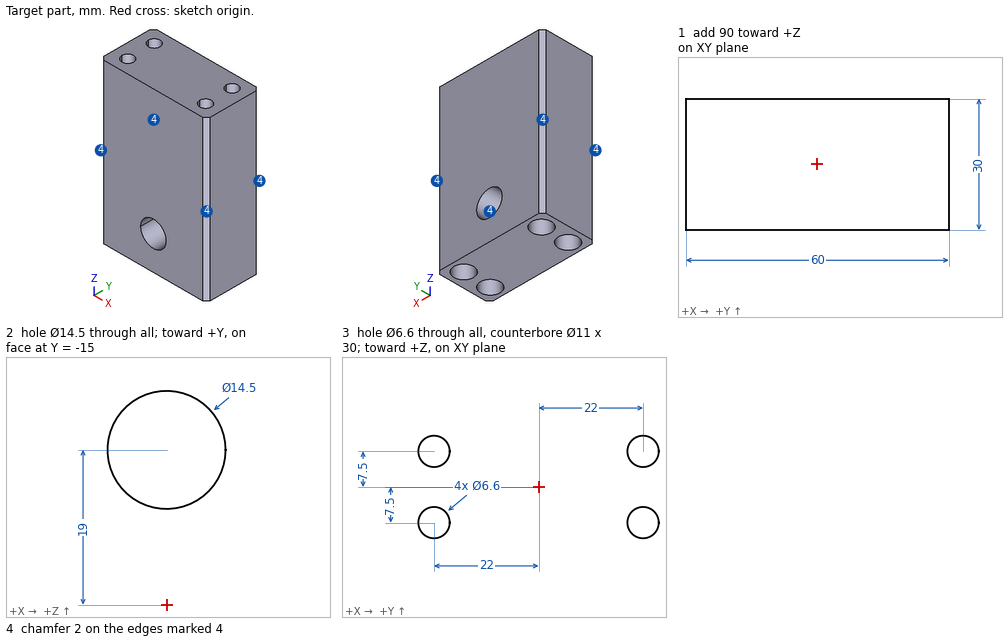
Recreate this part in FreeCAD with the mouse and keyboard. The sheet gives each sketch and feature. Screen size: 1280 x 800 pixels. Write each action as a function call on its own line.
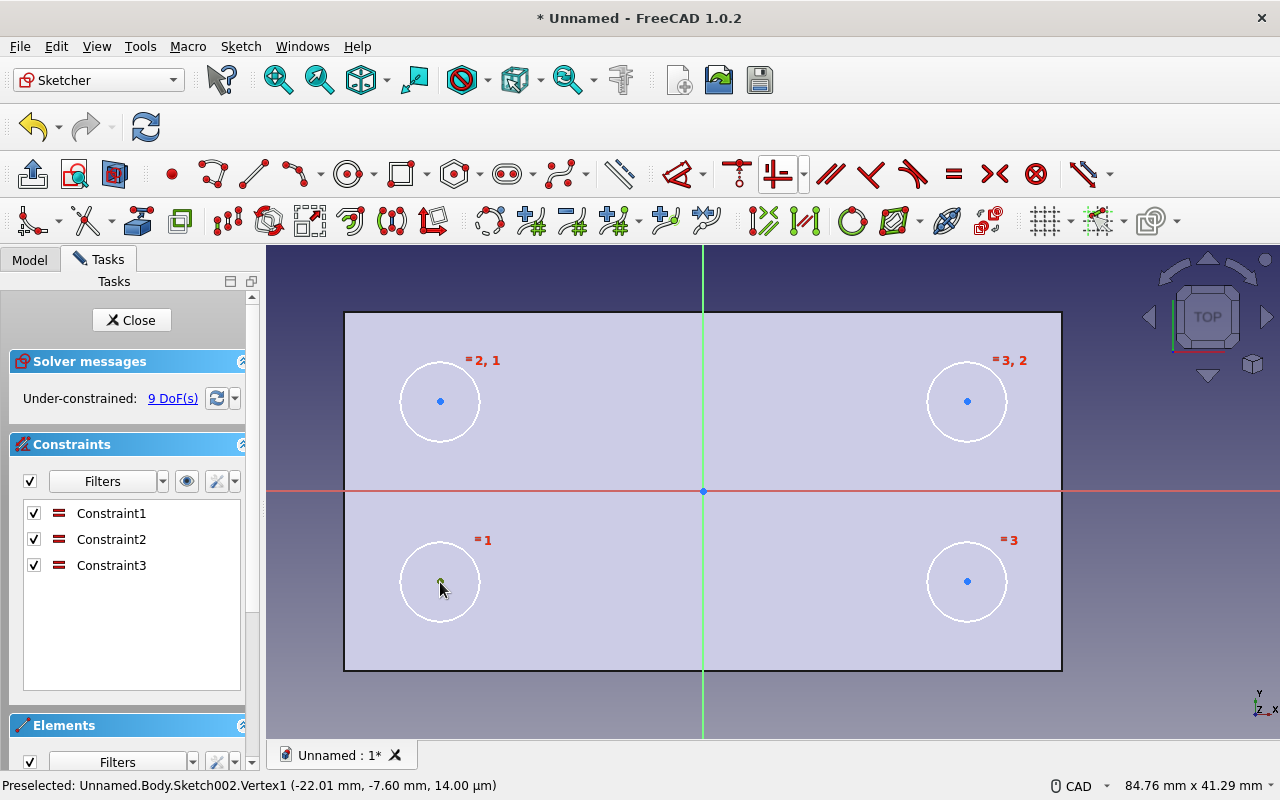
click(440, 402)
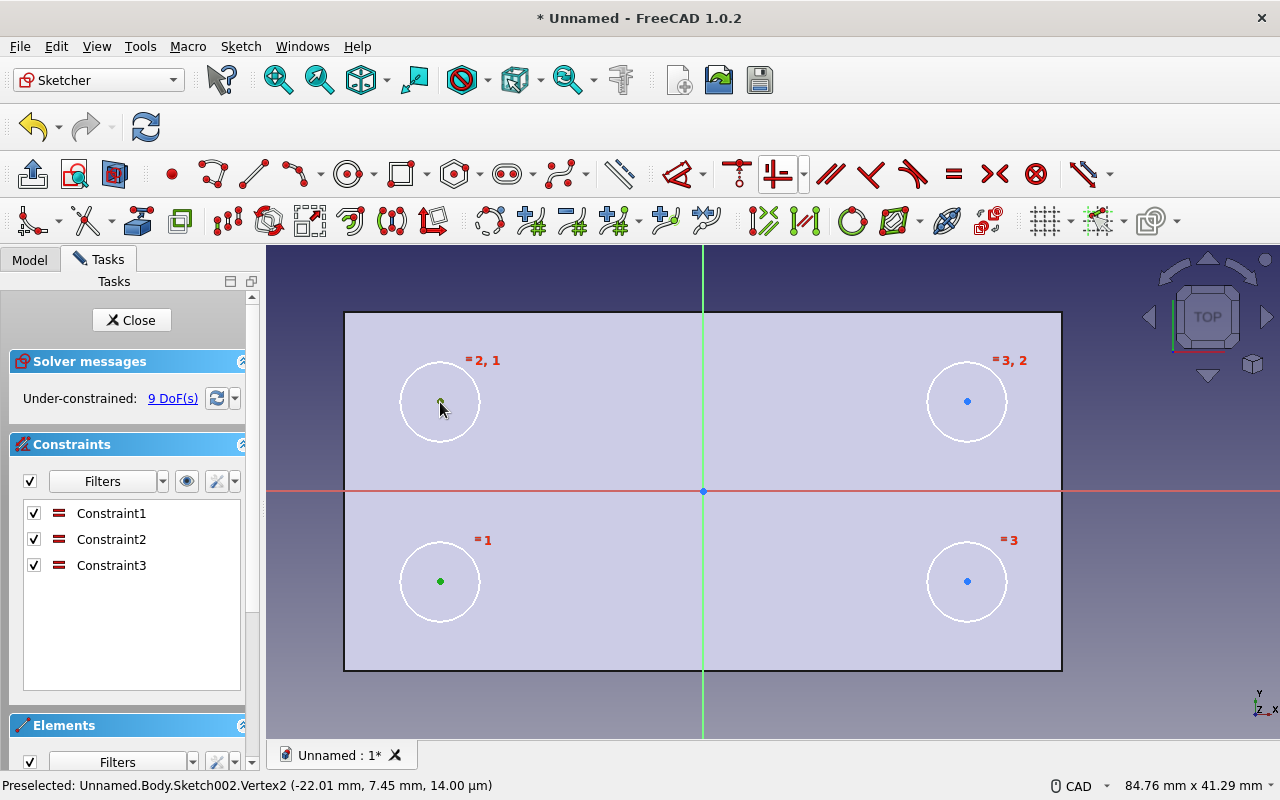
key(v)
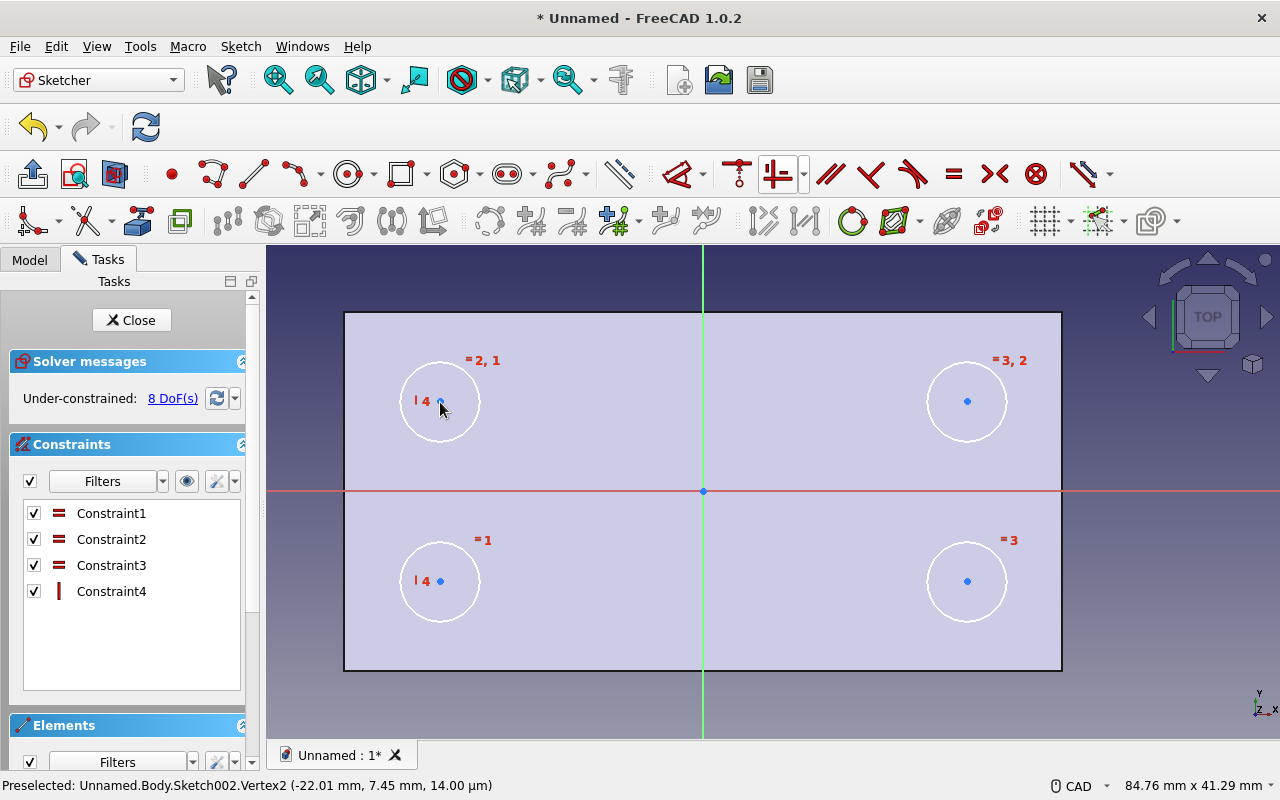
click(440, 402)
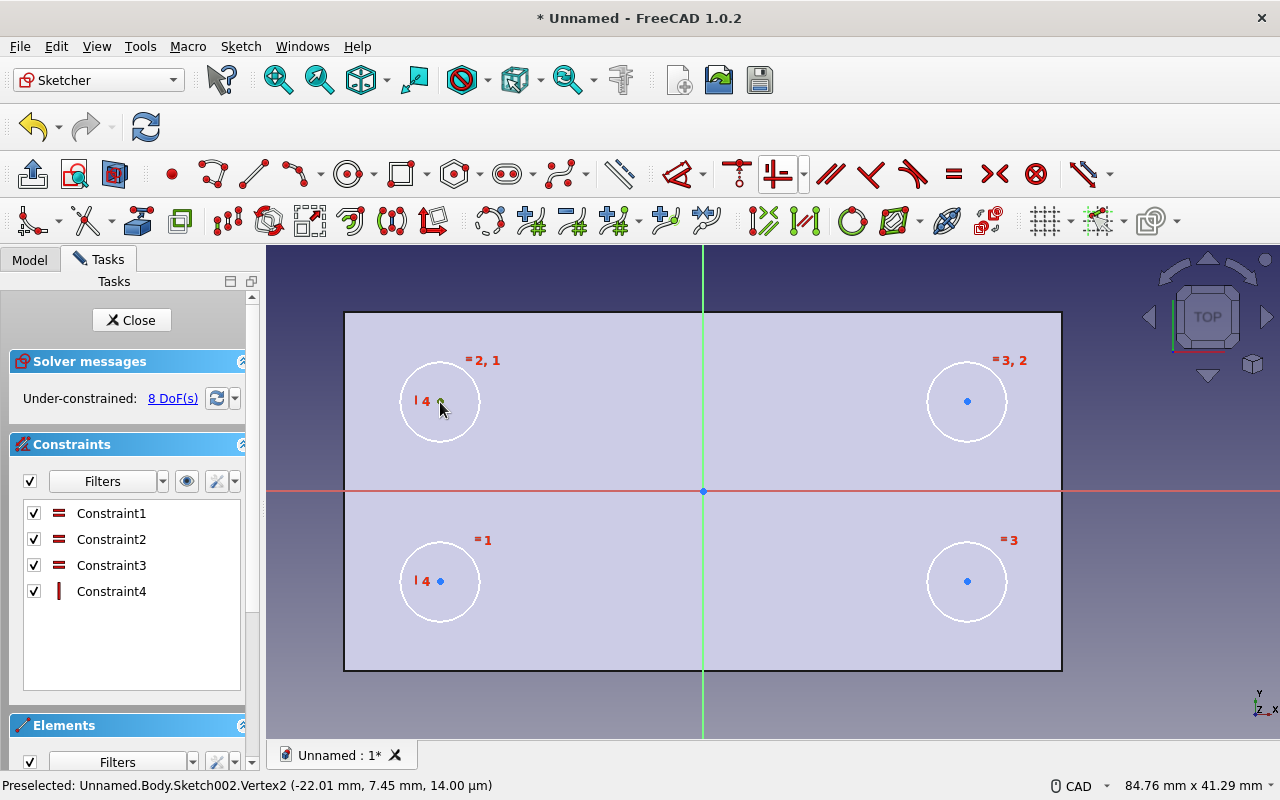
click(967, 402)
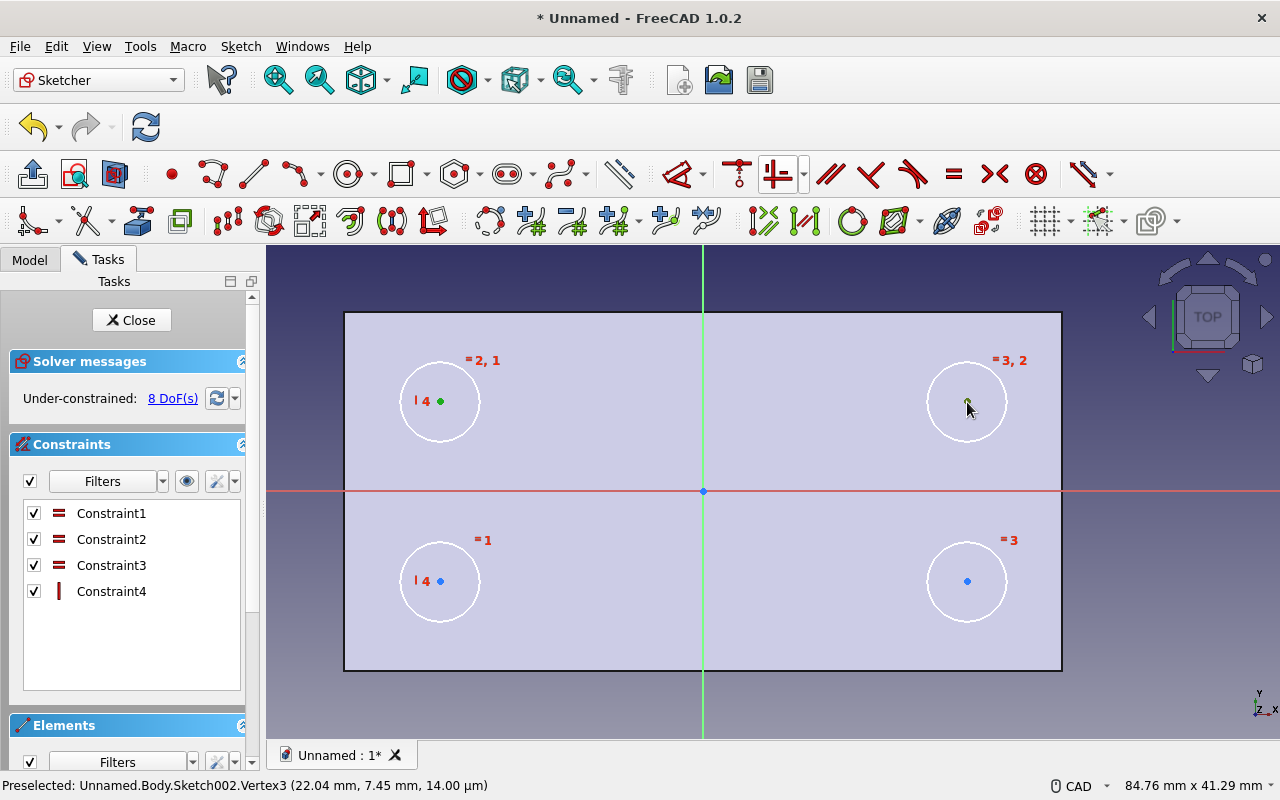
click(804, 174)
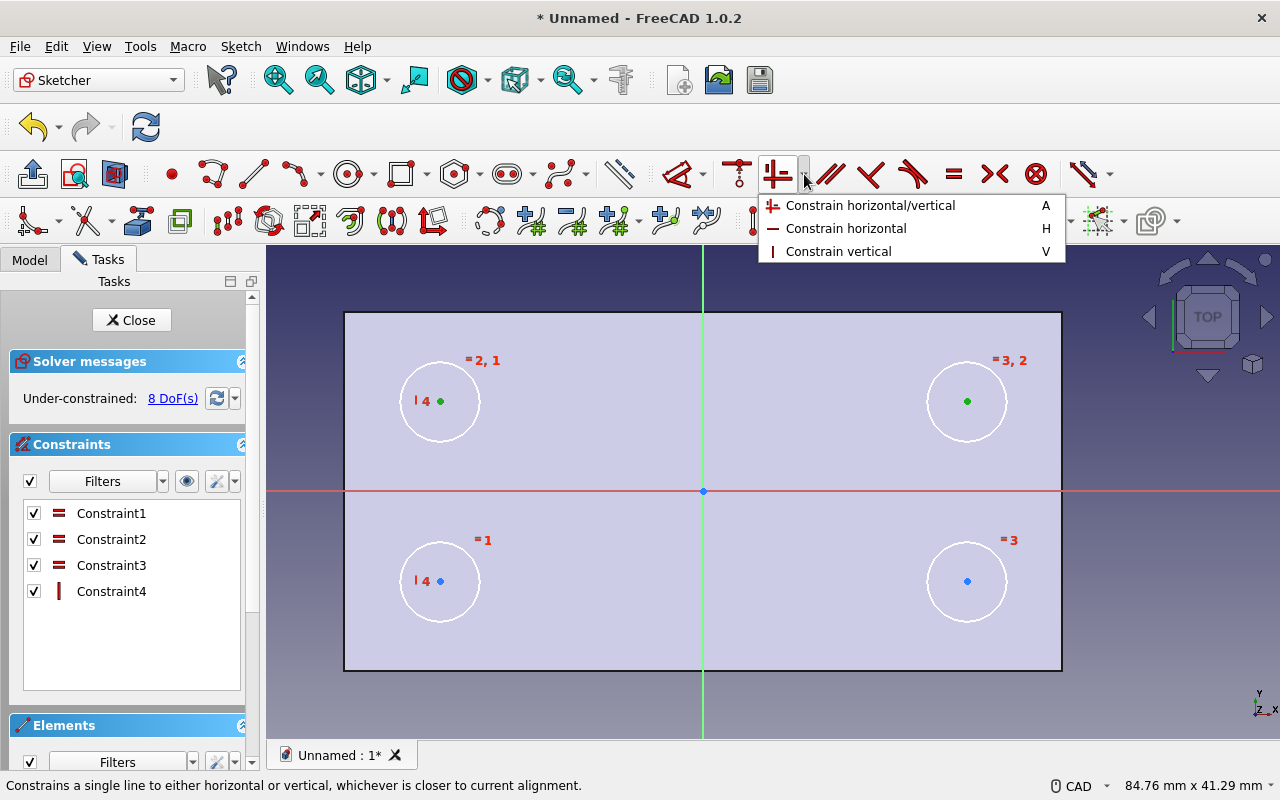
click(912, 228)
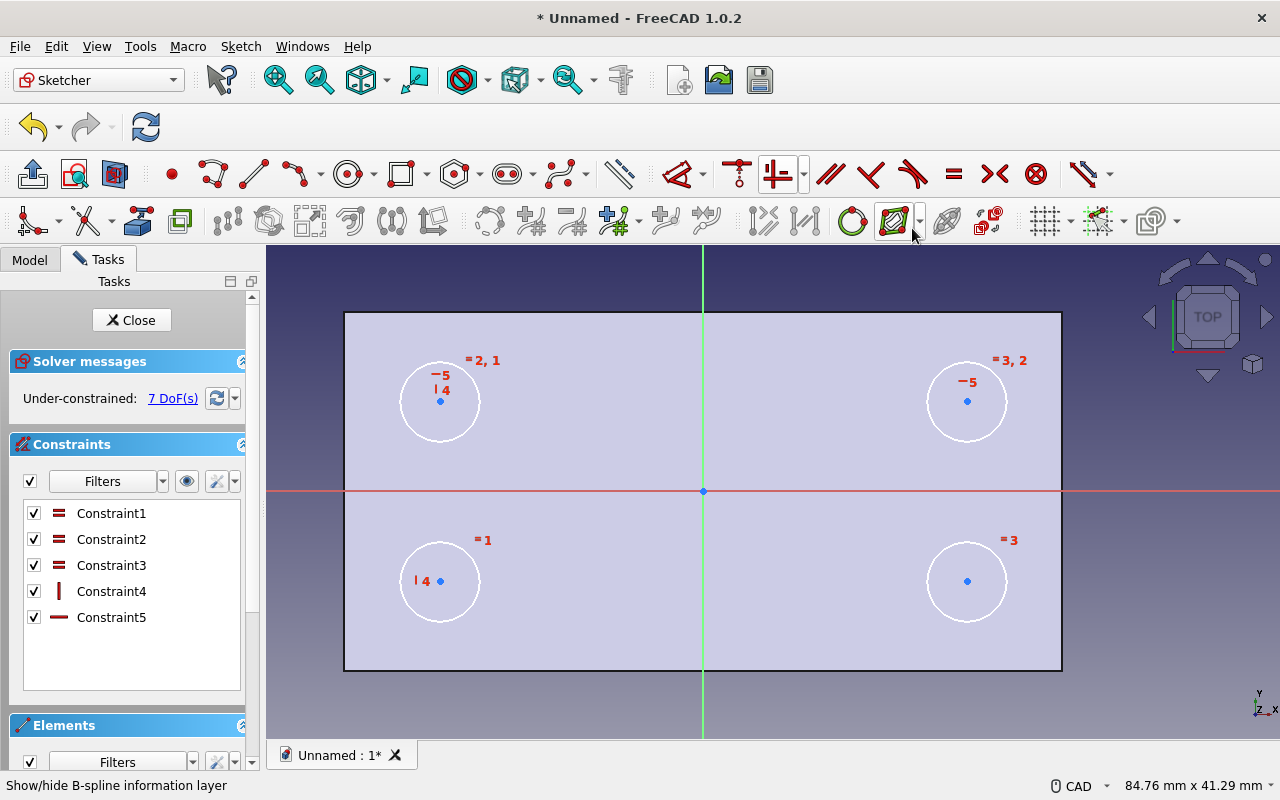
click(967, 402)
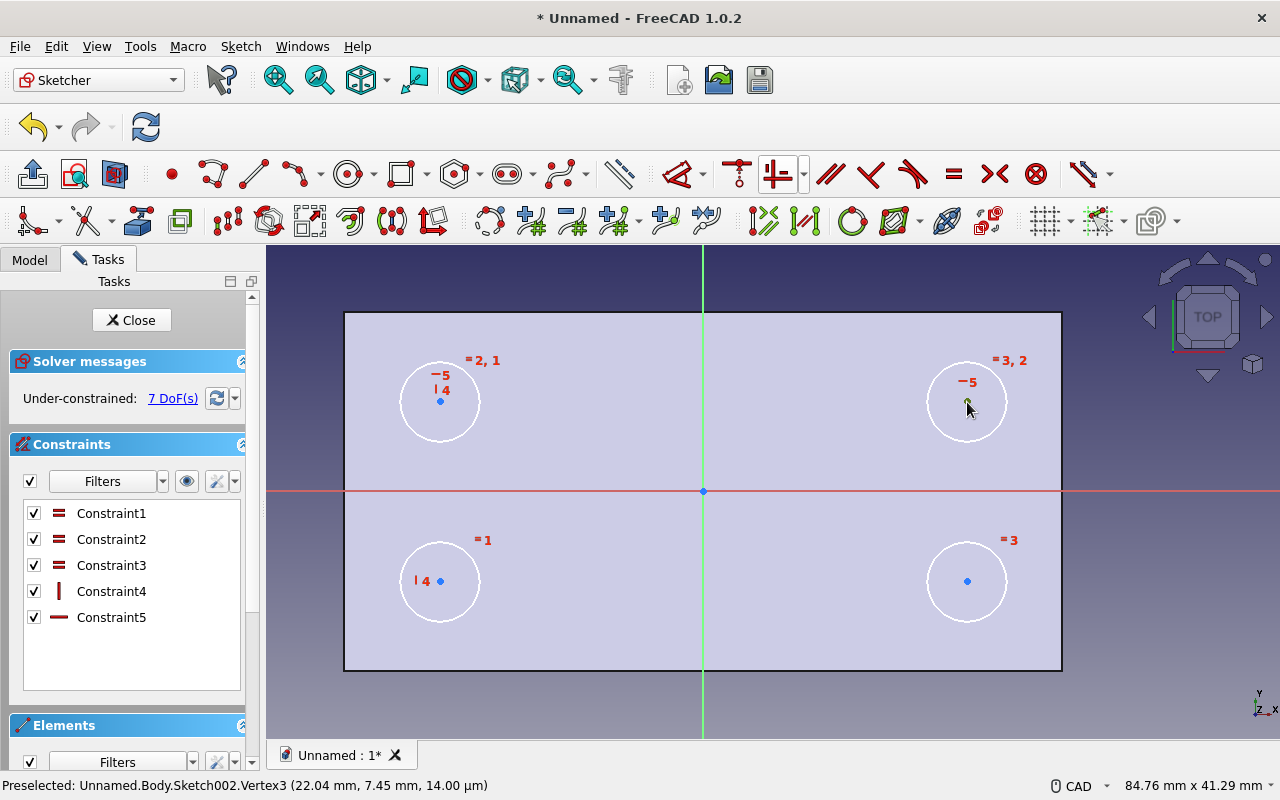
click(967, 582)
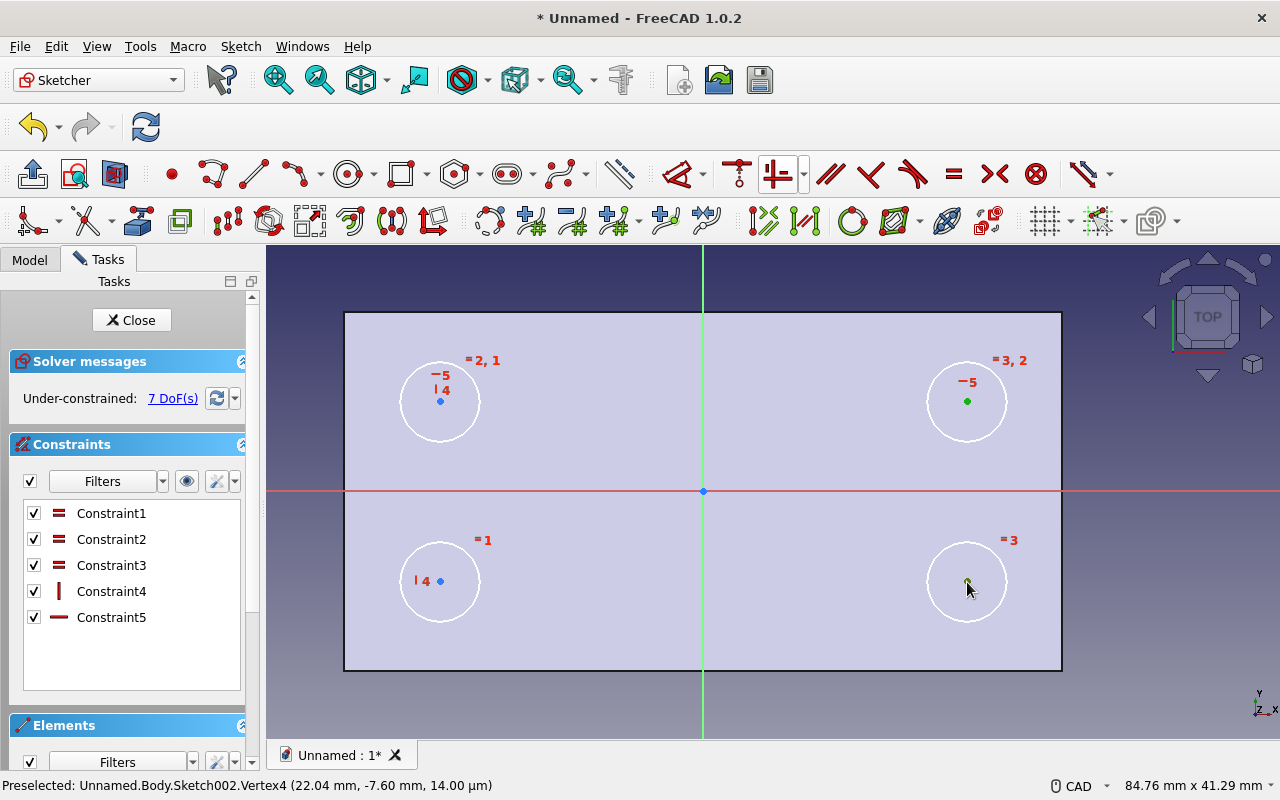
key(v)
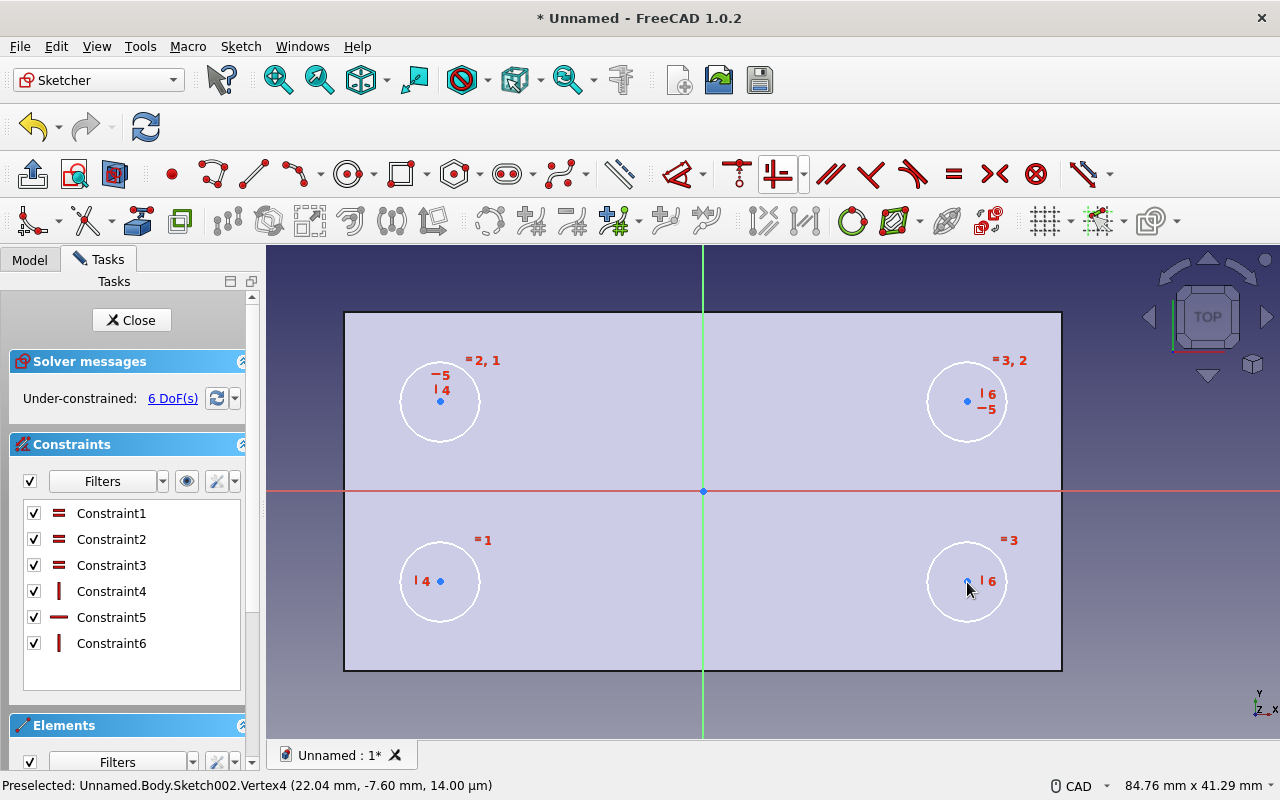
click(440, 582)